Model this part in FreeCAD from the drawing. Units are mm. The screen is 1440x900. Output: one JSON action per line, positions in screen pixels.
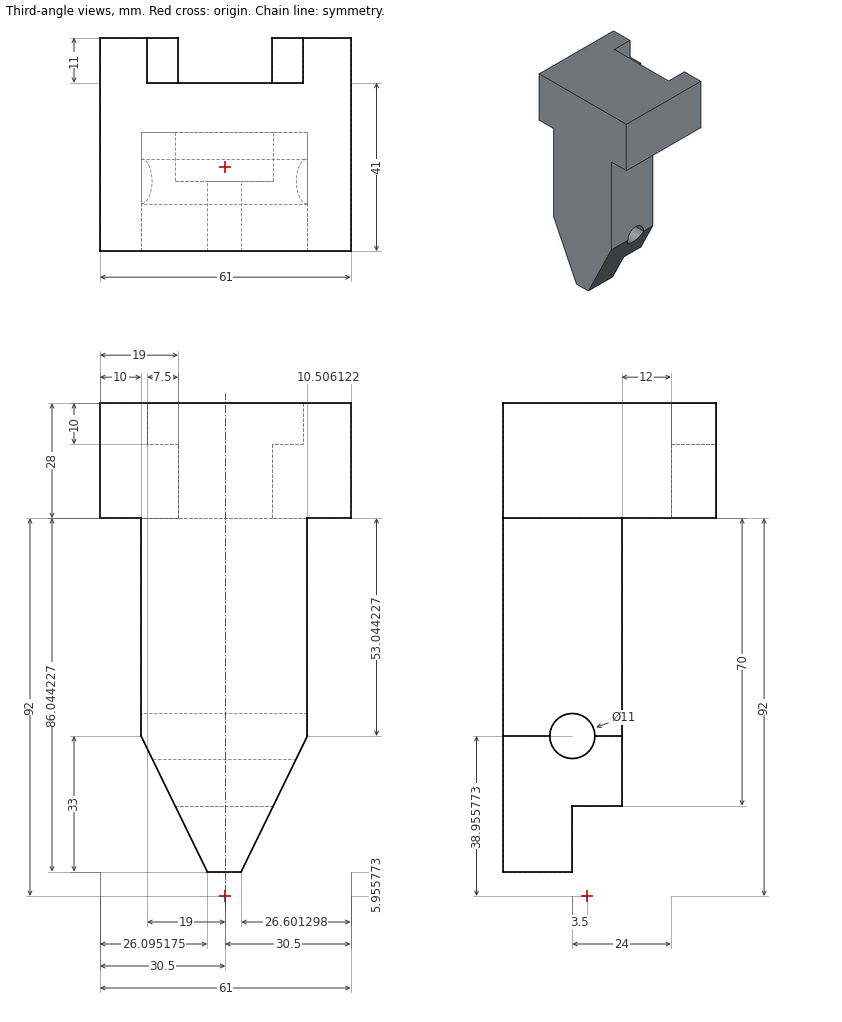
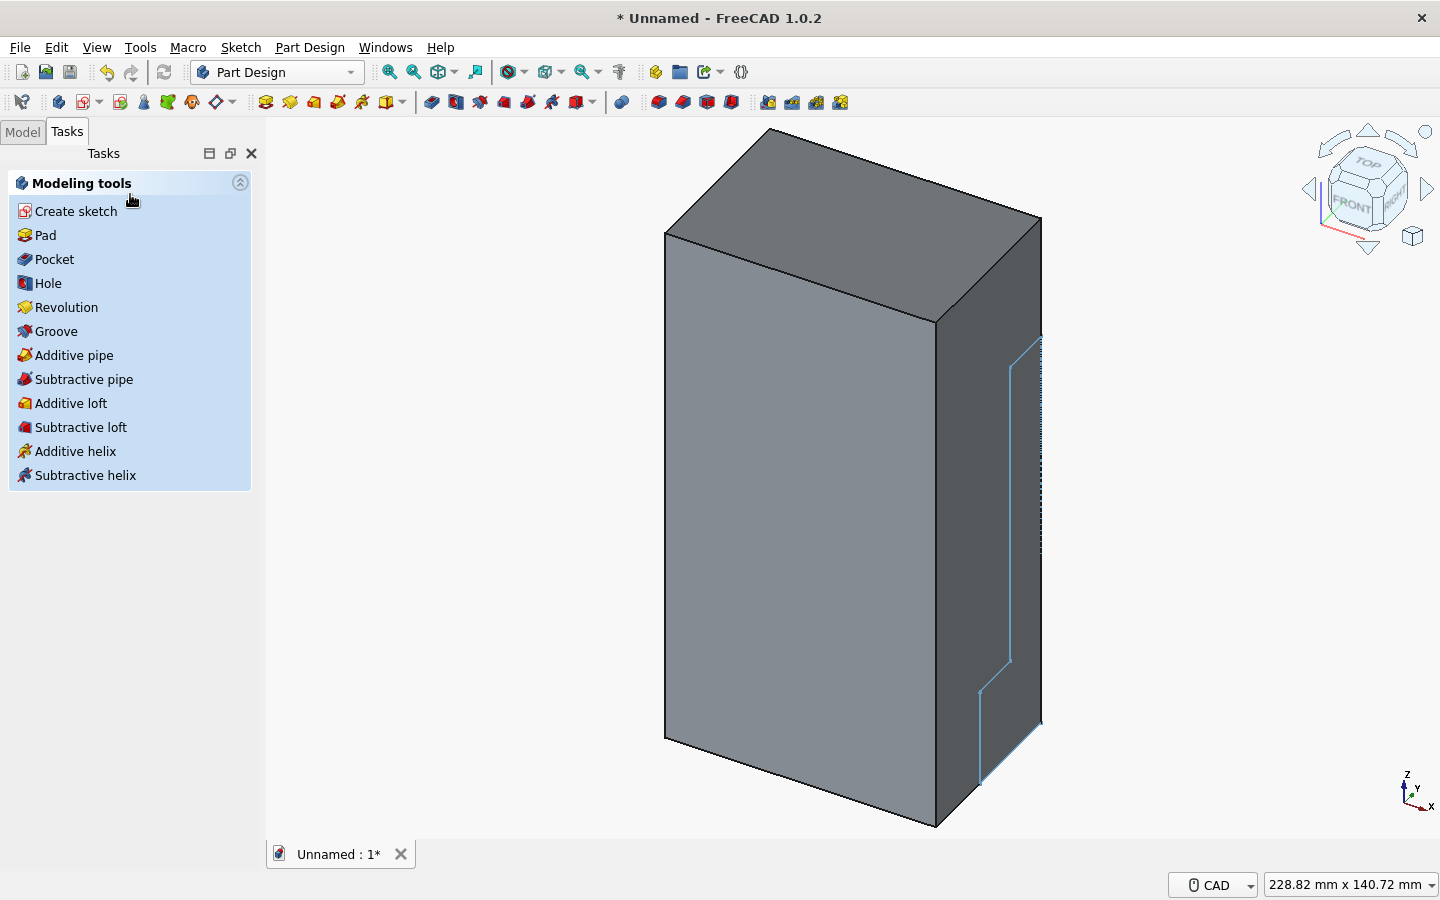
{"action": "left_click", "coordinate": [432, 102]}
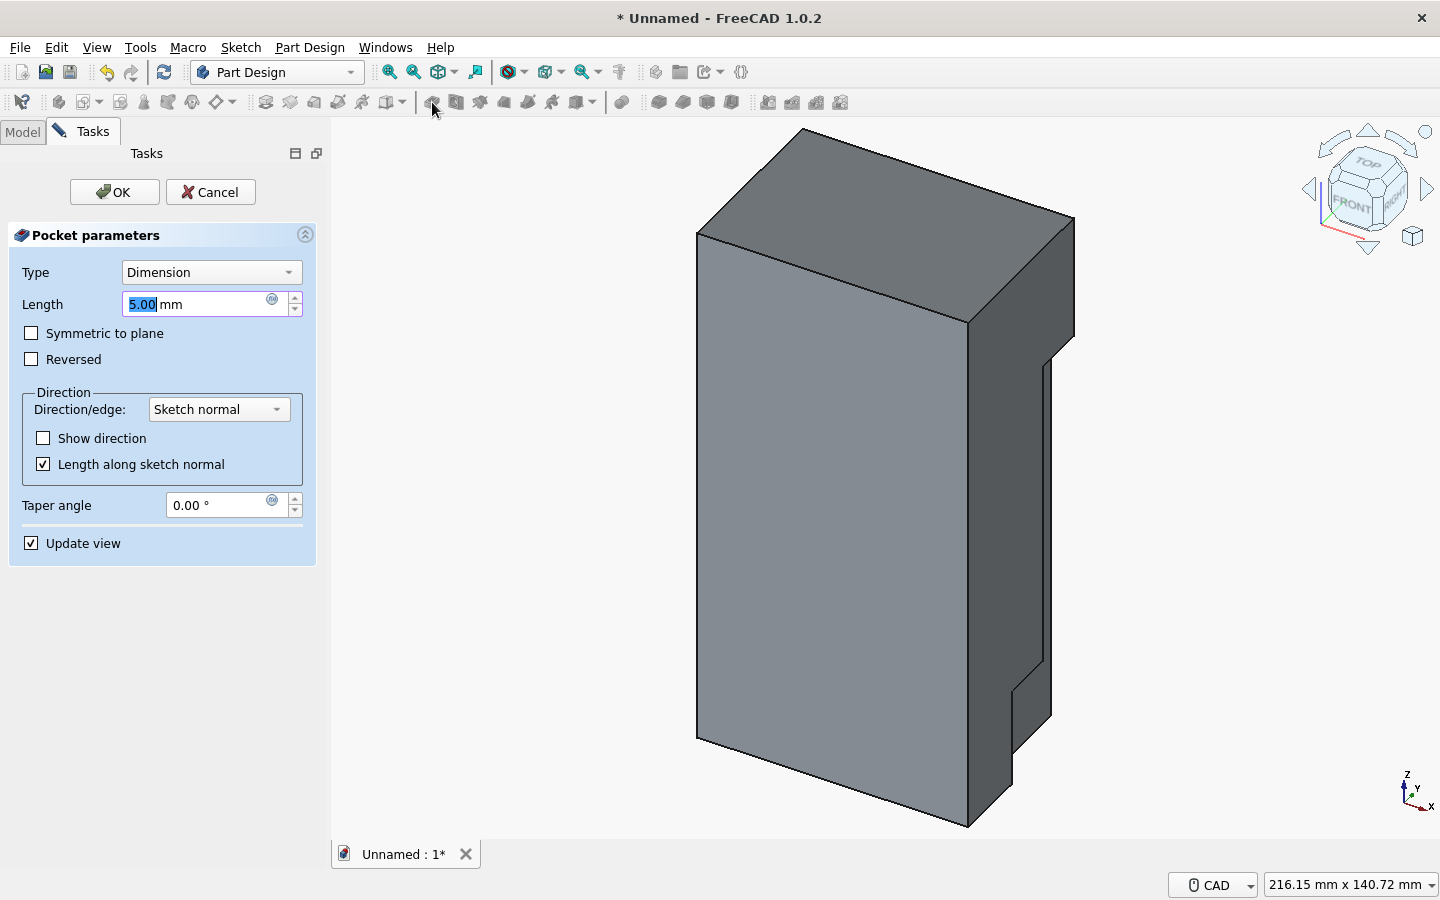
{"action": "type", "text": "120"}
{"action": "key", "text": "Tab"}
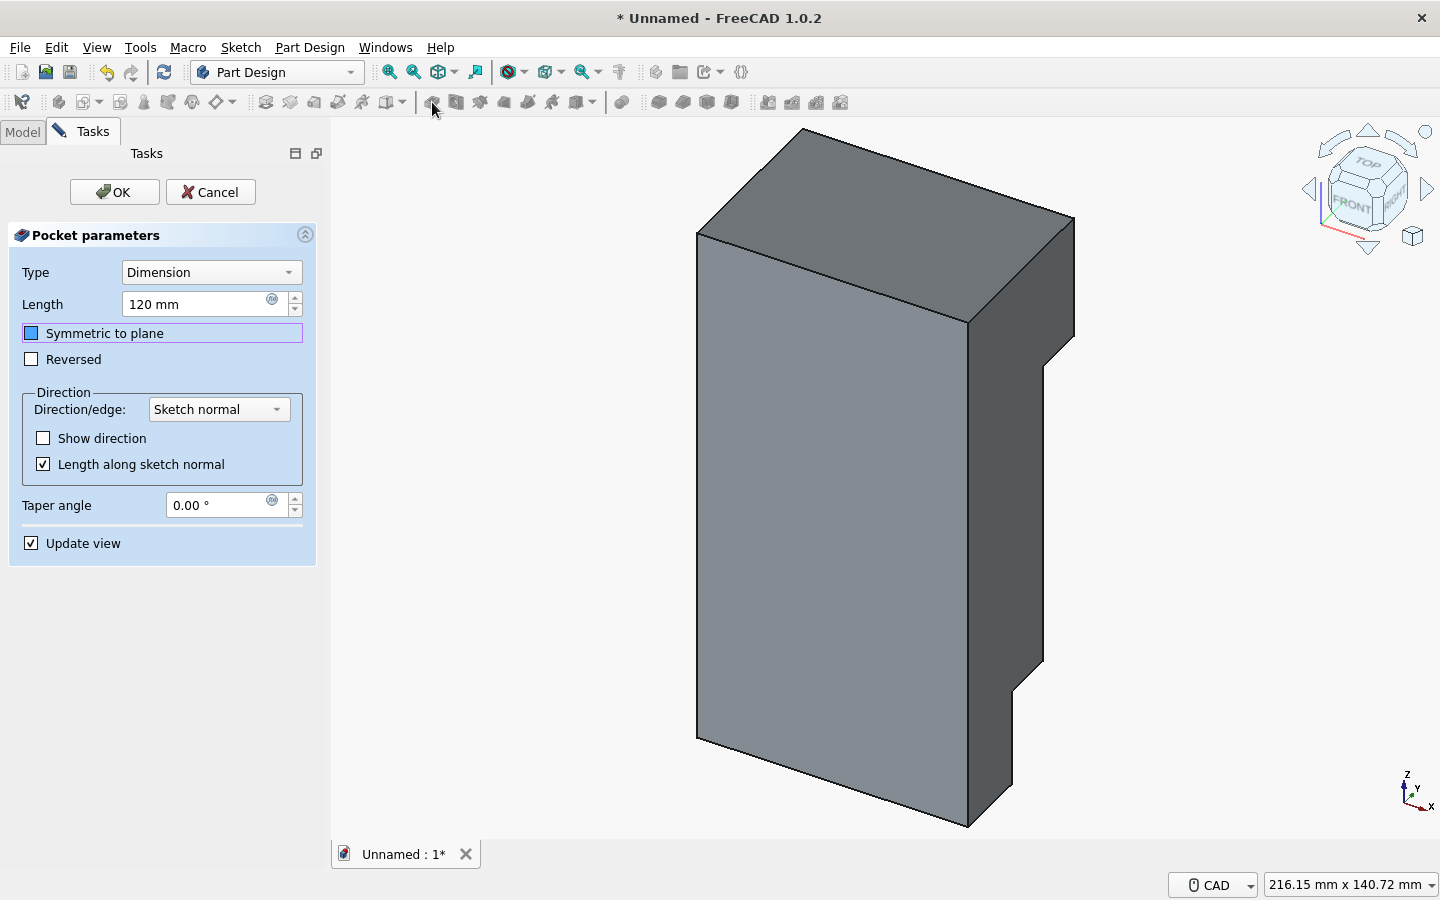
{"action": "left_click", "coordinate": [115, 192]}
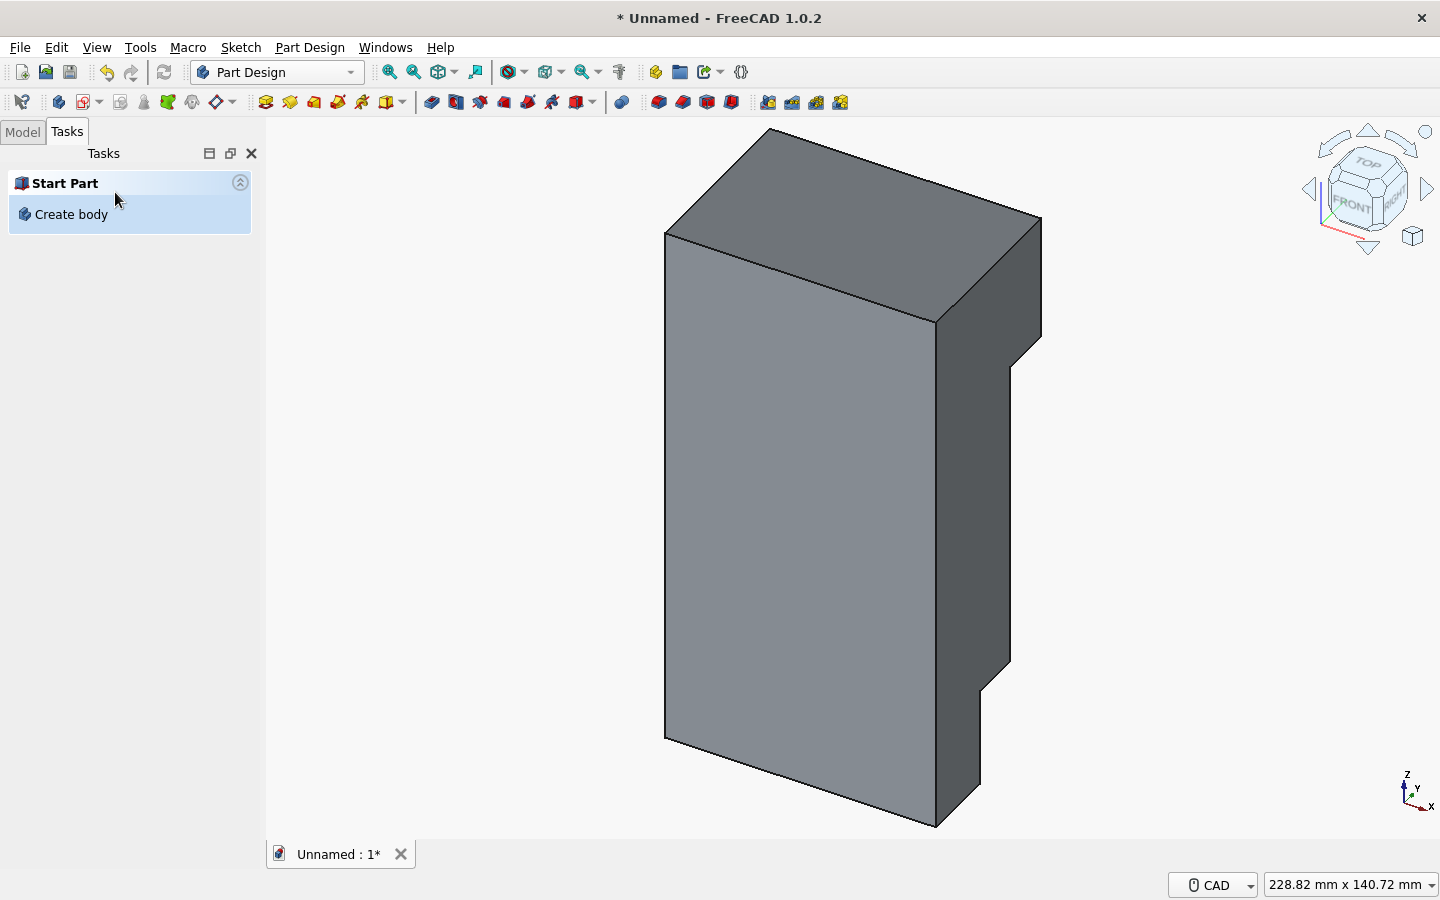
{"action": "key", "text": "4"}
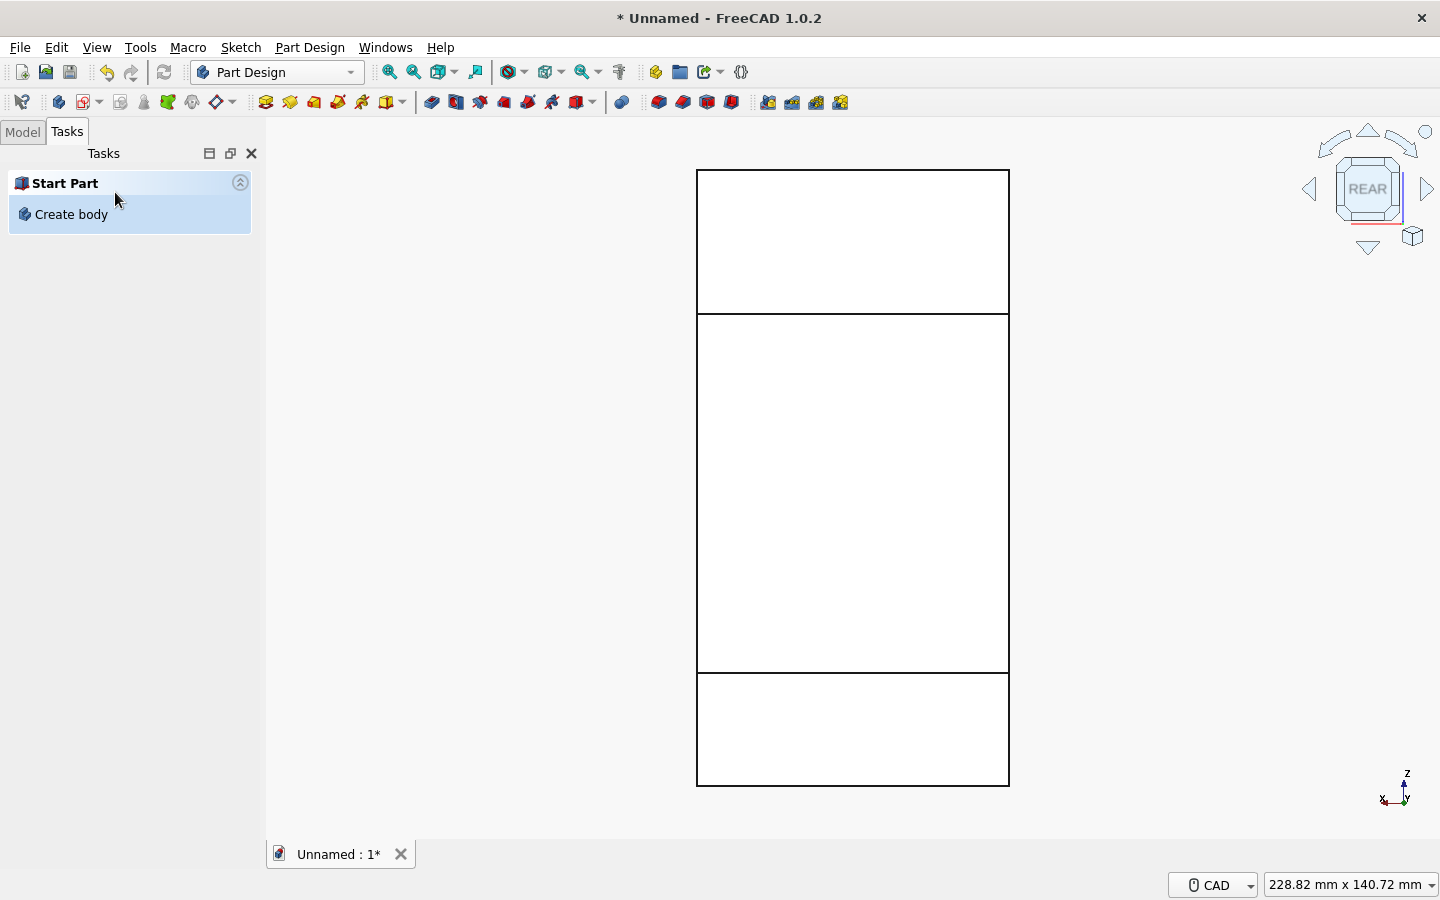
{"action": "left_click", "coordinate": [808, 241]}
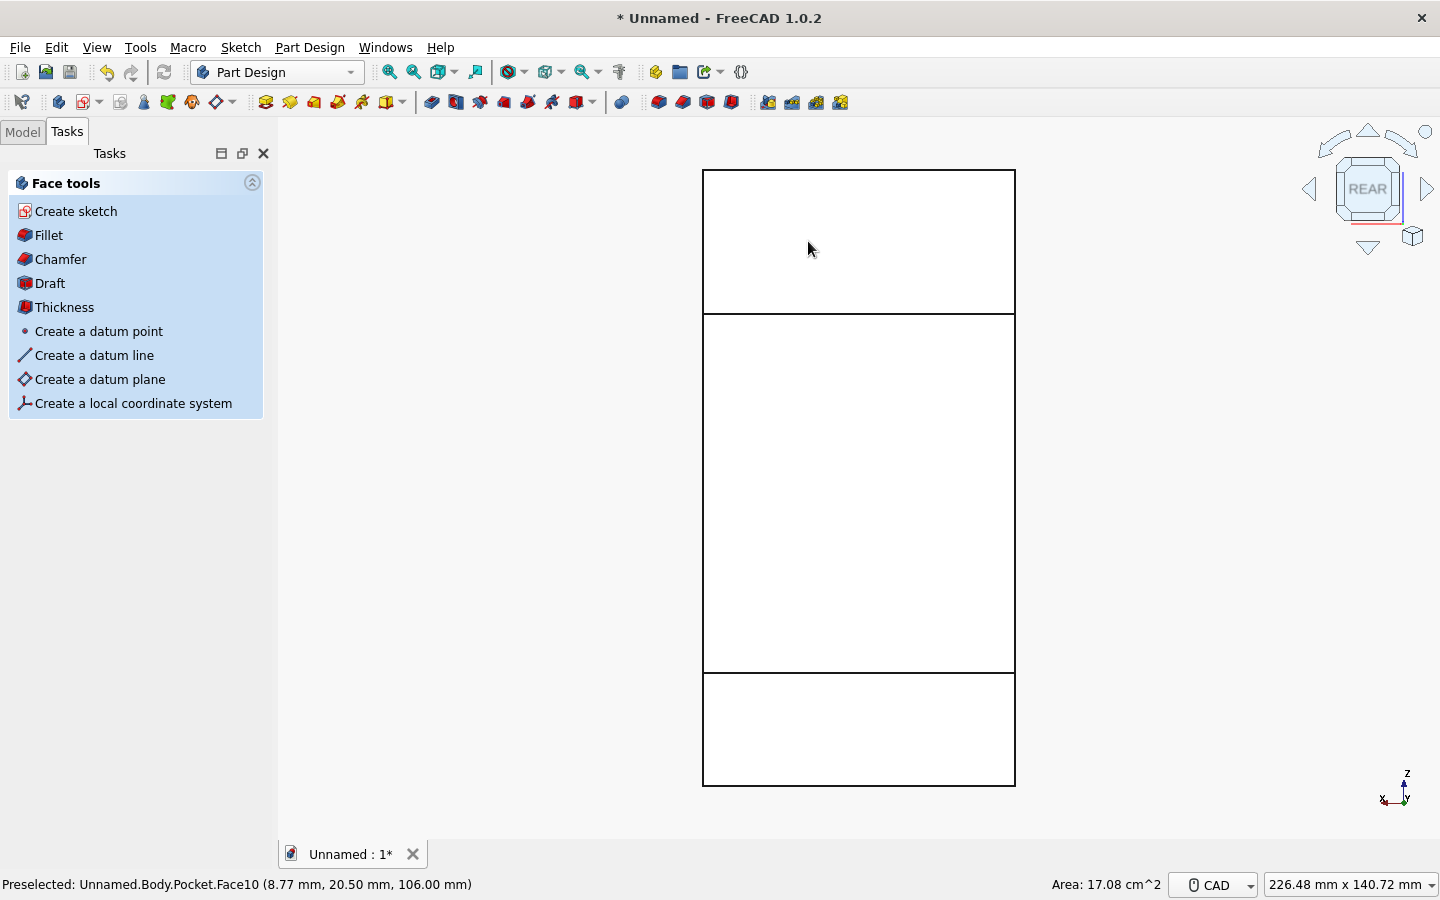
{"action": "left_click", "coordinate": [84, 102]}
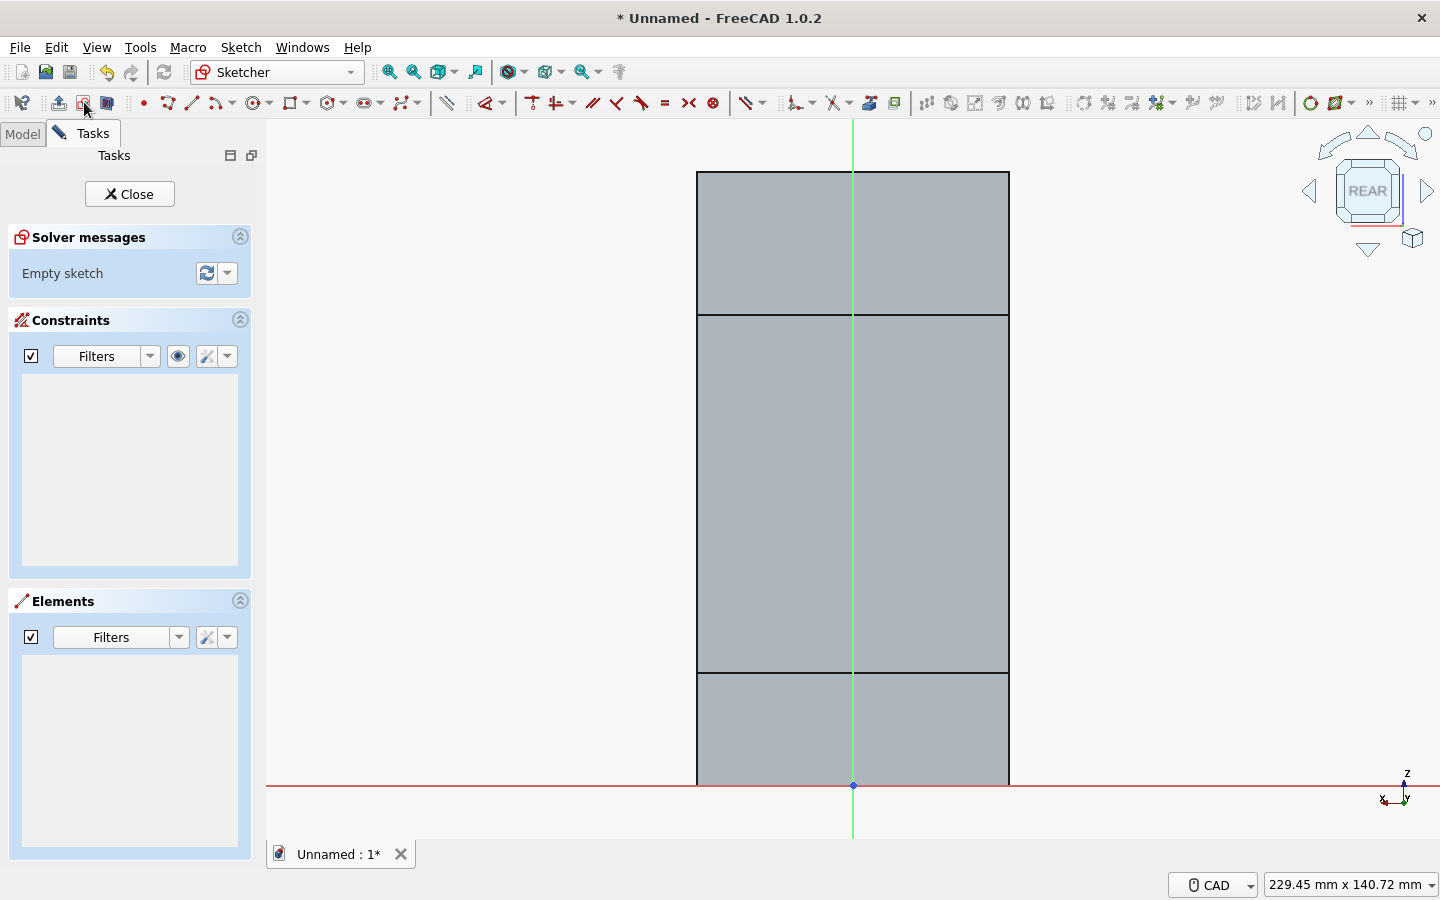
{"action": "left_click", "coordinate": [168, 104]}